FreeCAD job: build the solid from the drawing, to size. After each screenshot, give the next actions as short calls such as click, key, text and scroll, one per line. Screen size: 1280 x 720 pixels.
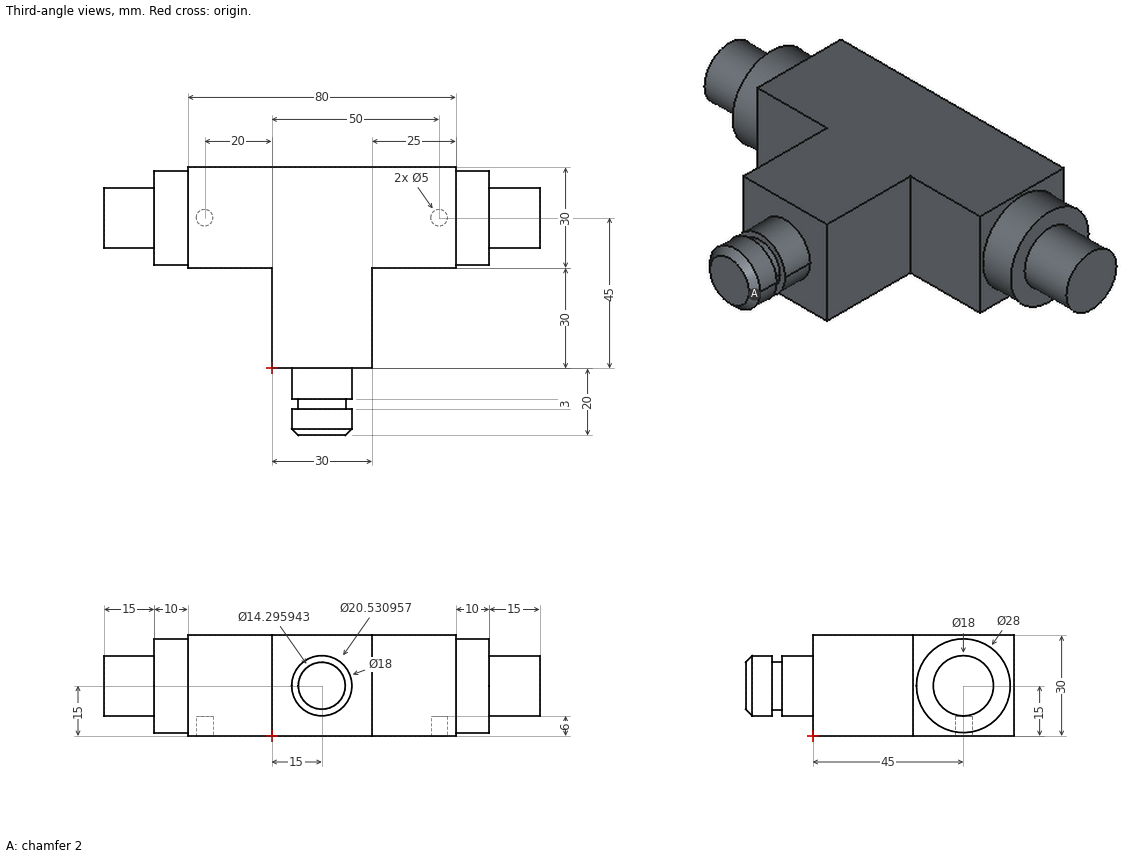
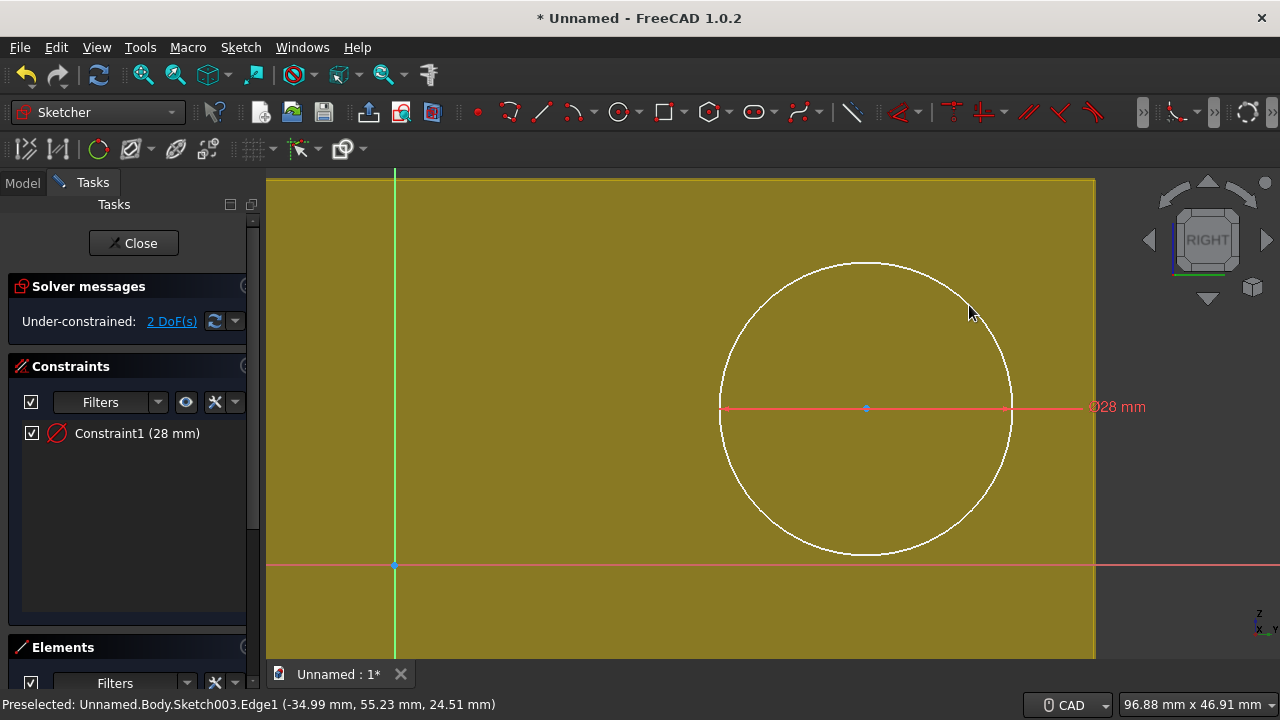
click(898, 112)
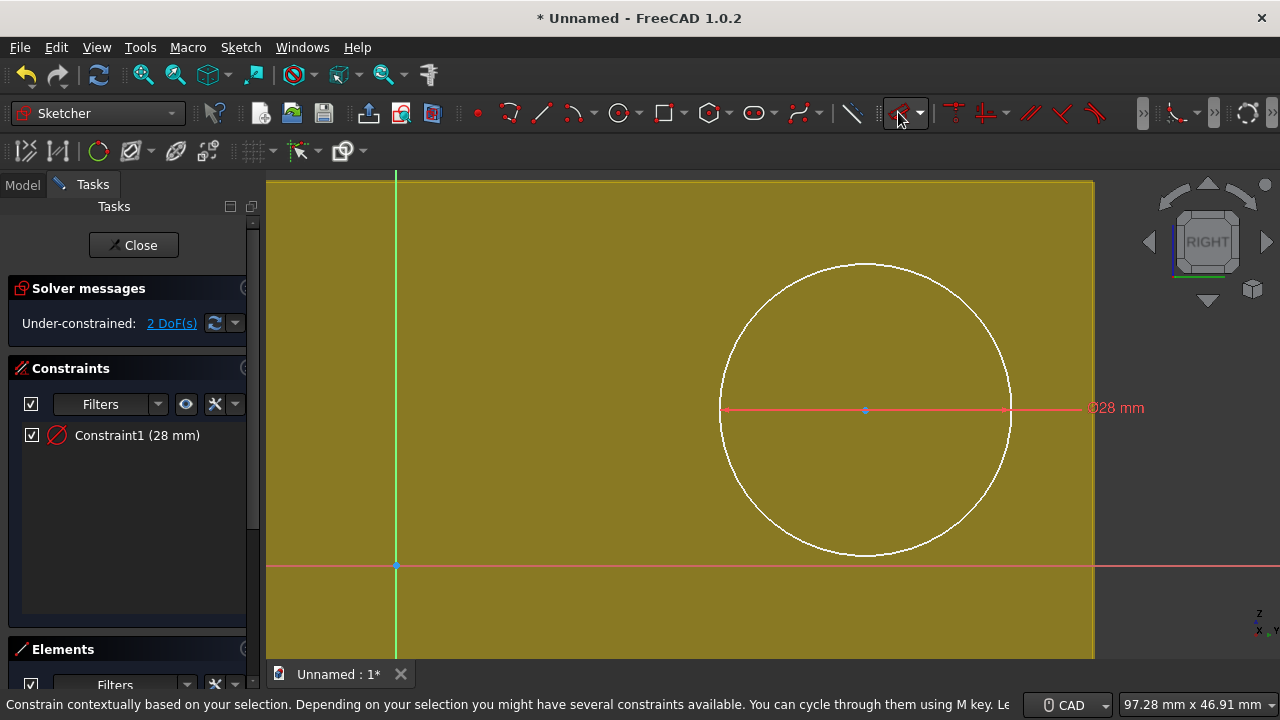
click(866, 410)
click(631, 600)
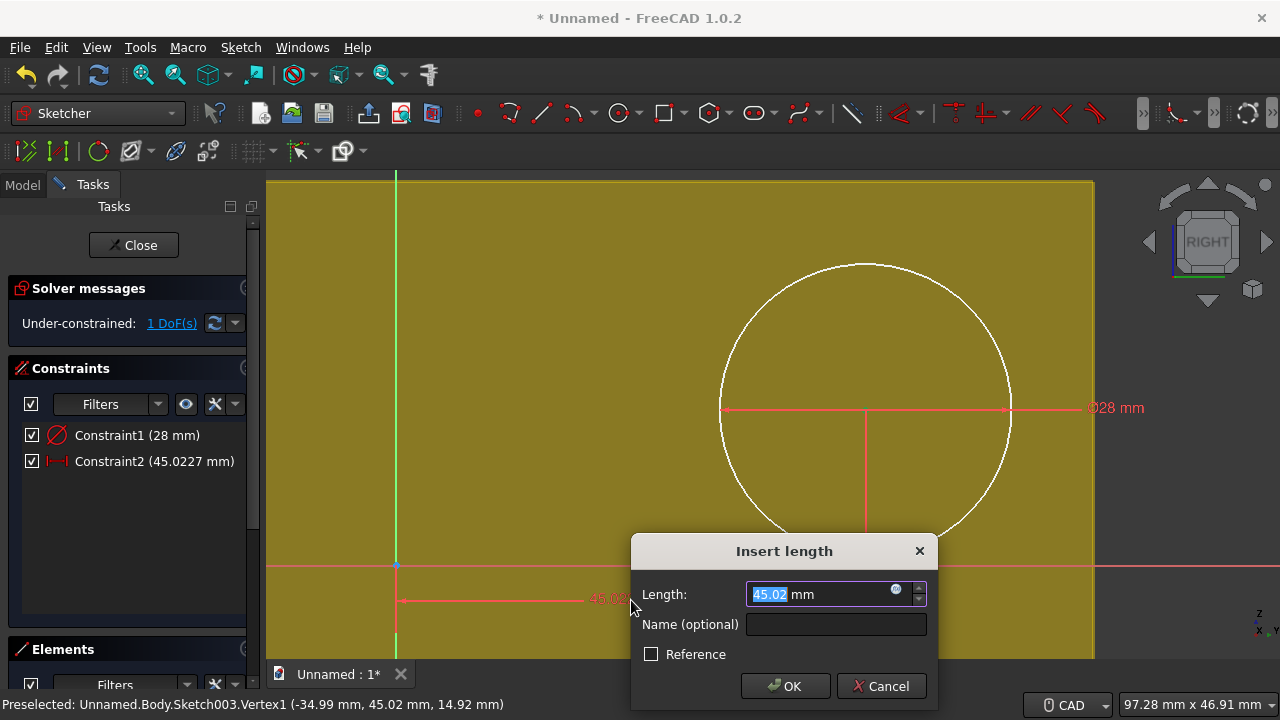
text(45)
key(Return)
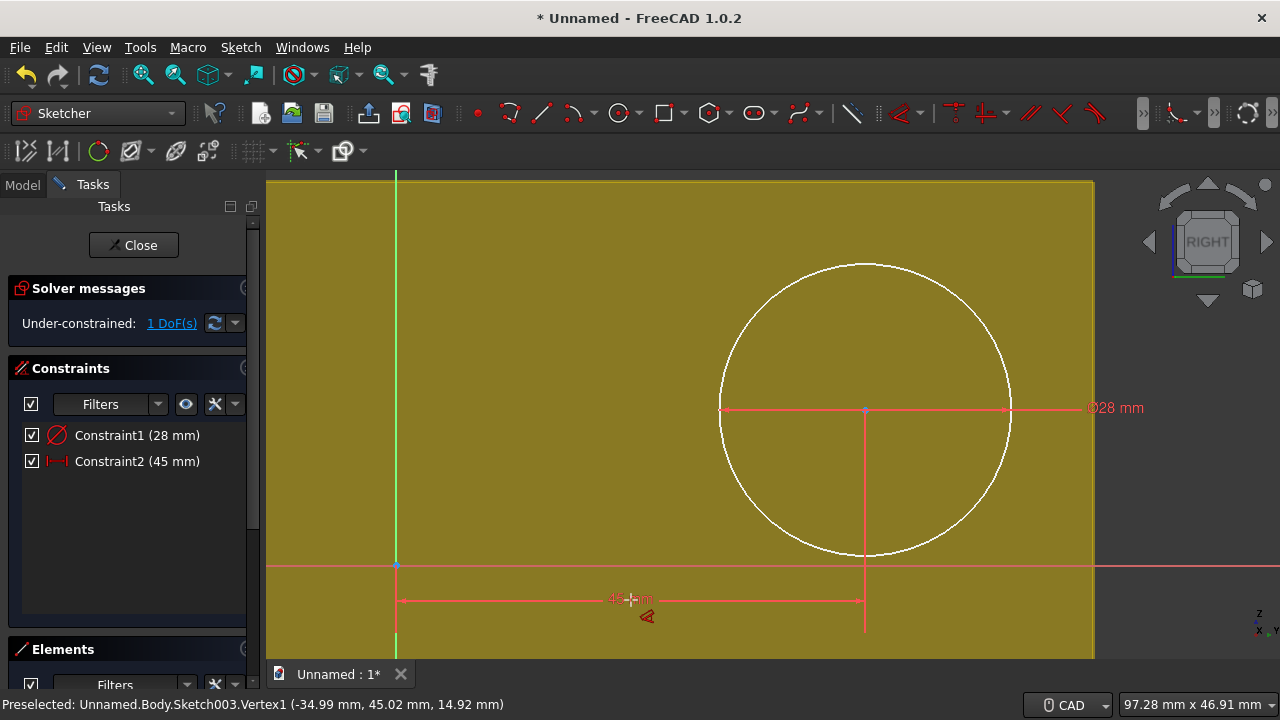
click(865, 410)
click(362, 488)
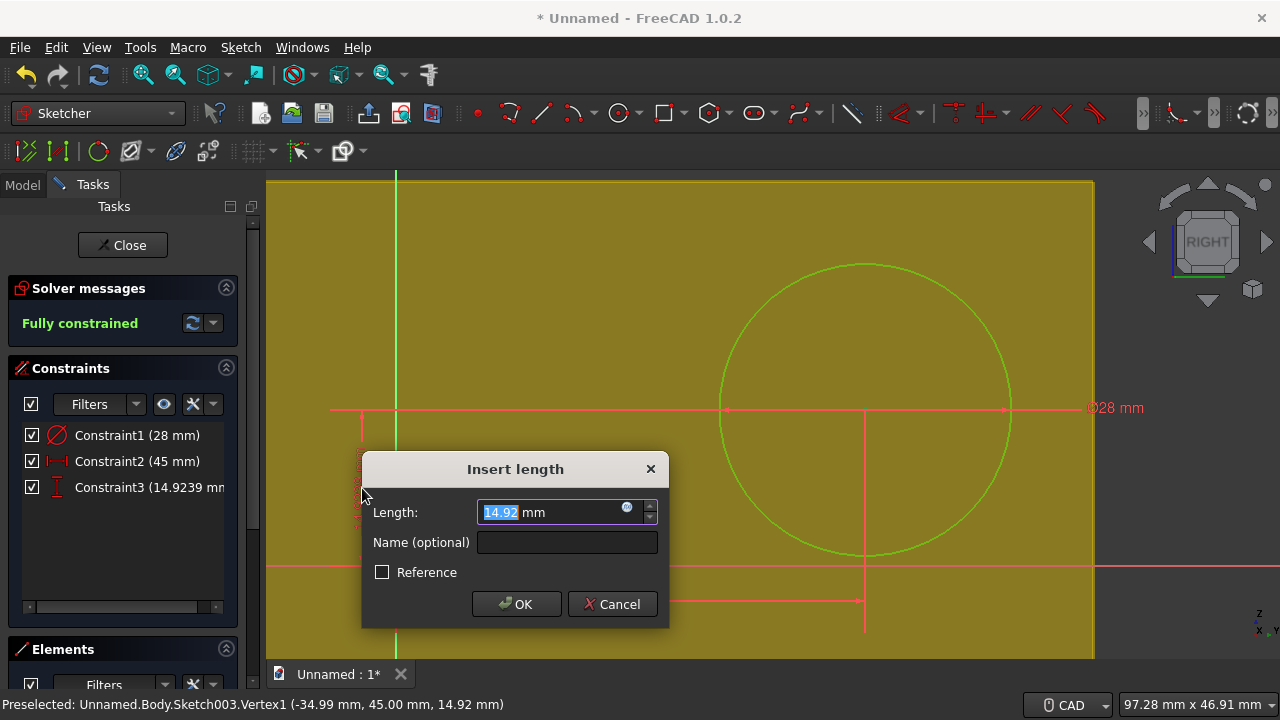
text(15)
key(Return)
key(Escape)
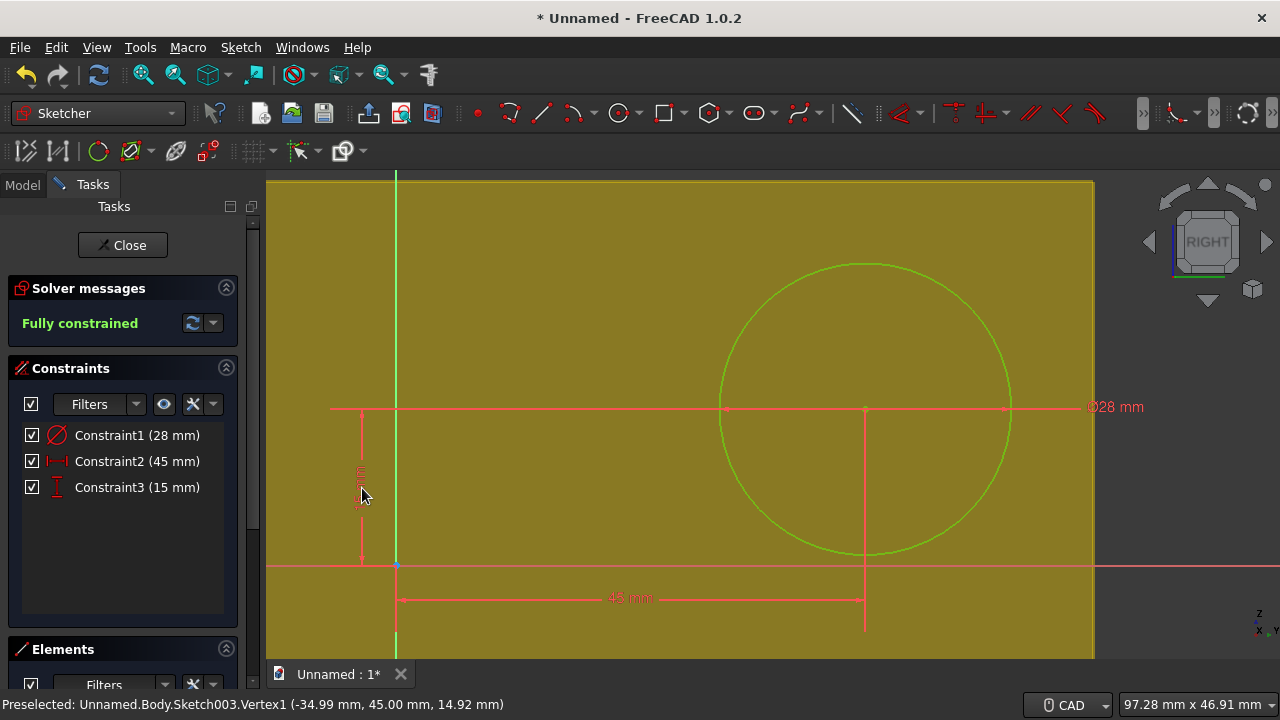
click(123, 245)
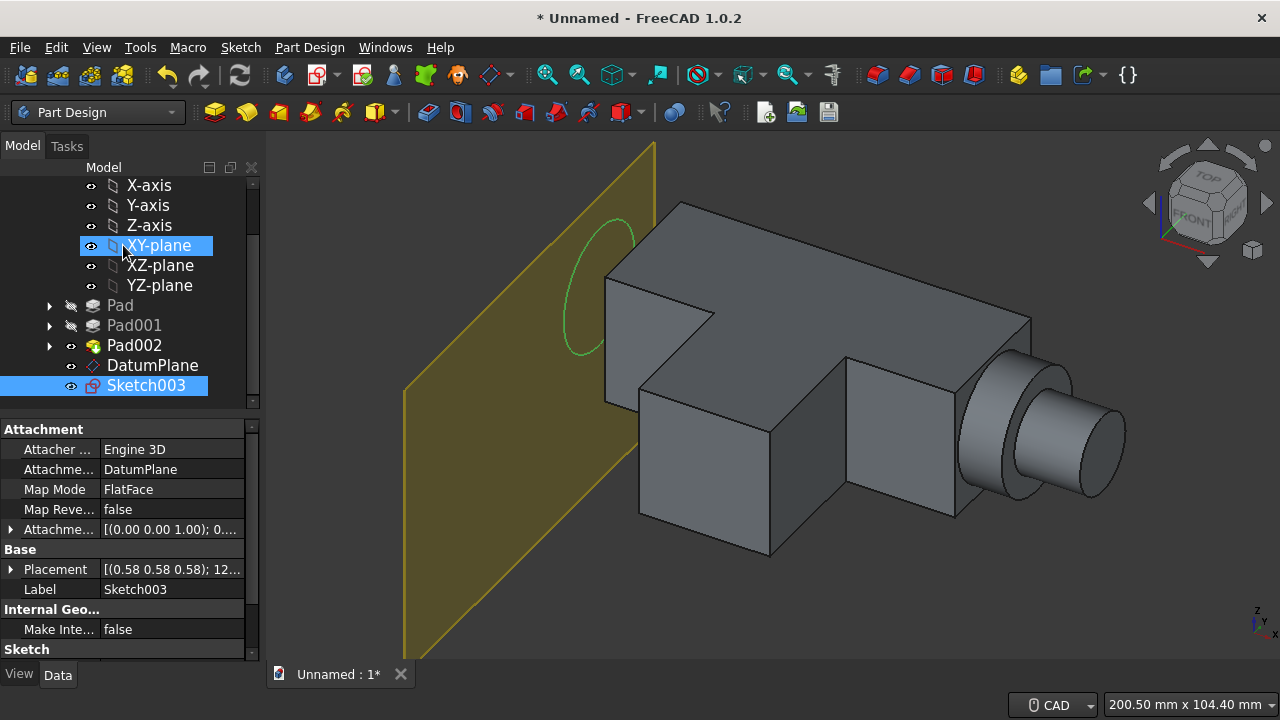
click(216, 112)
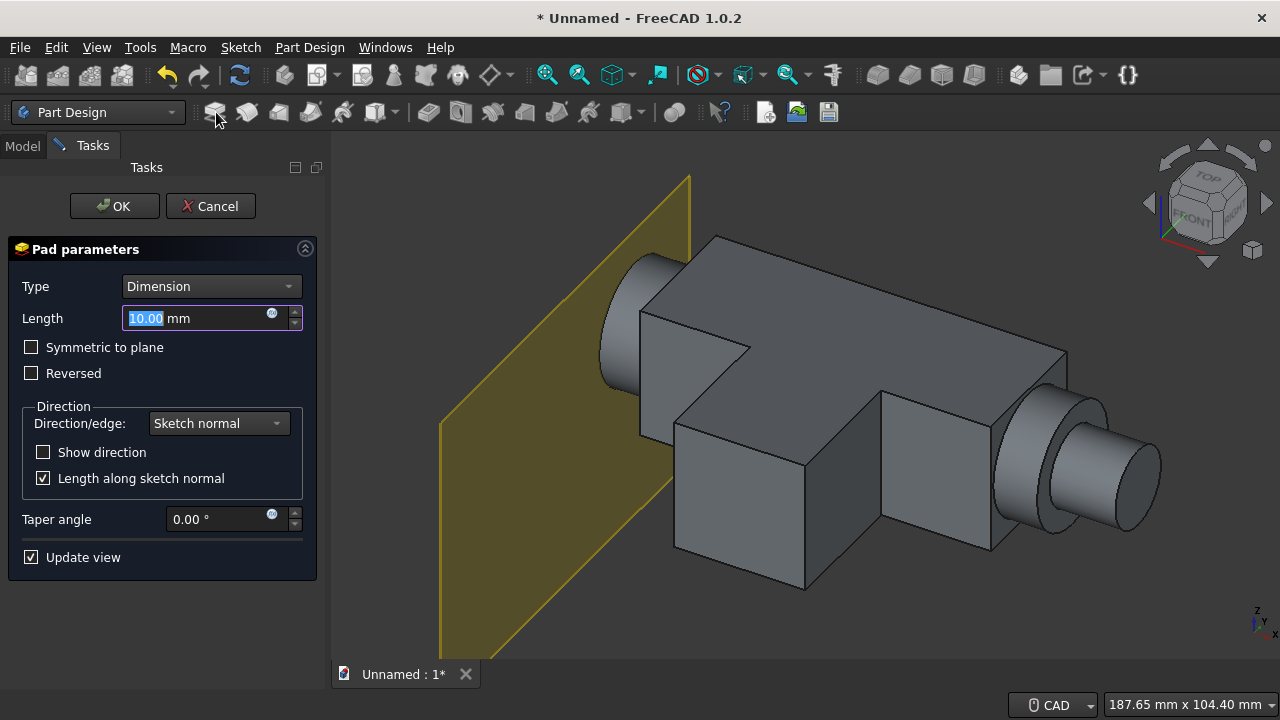
text(10)
key(Tab)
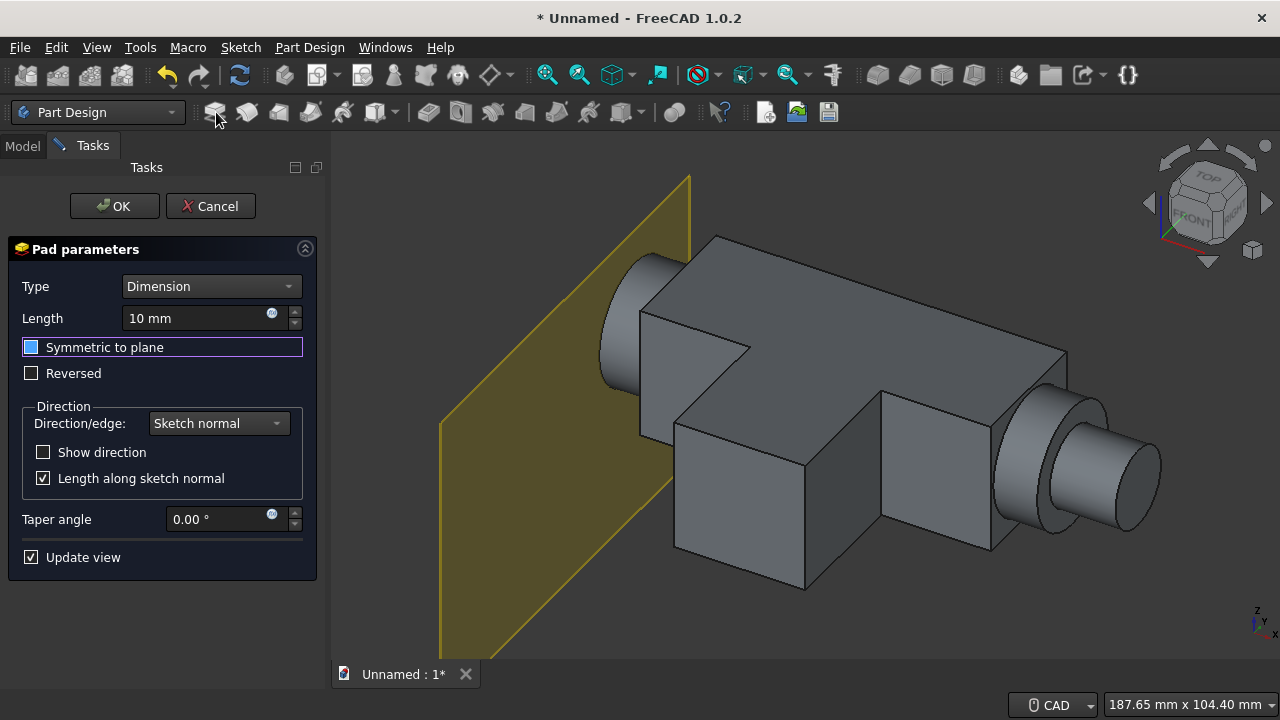
click(115, 206)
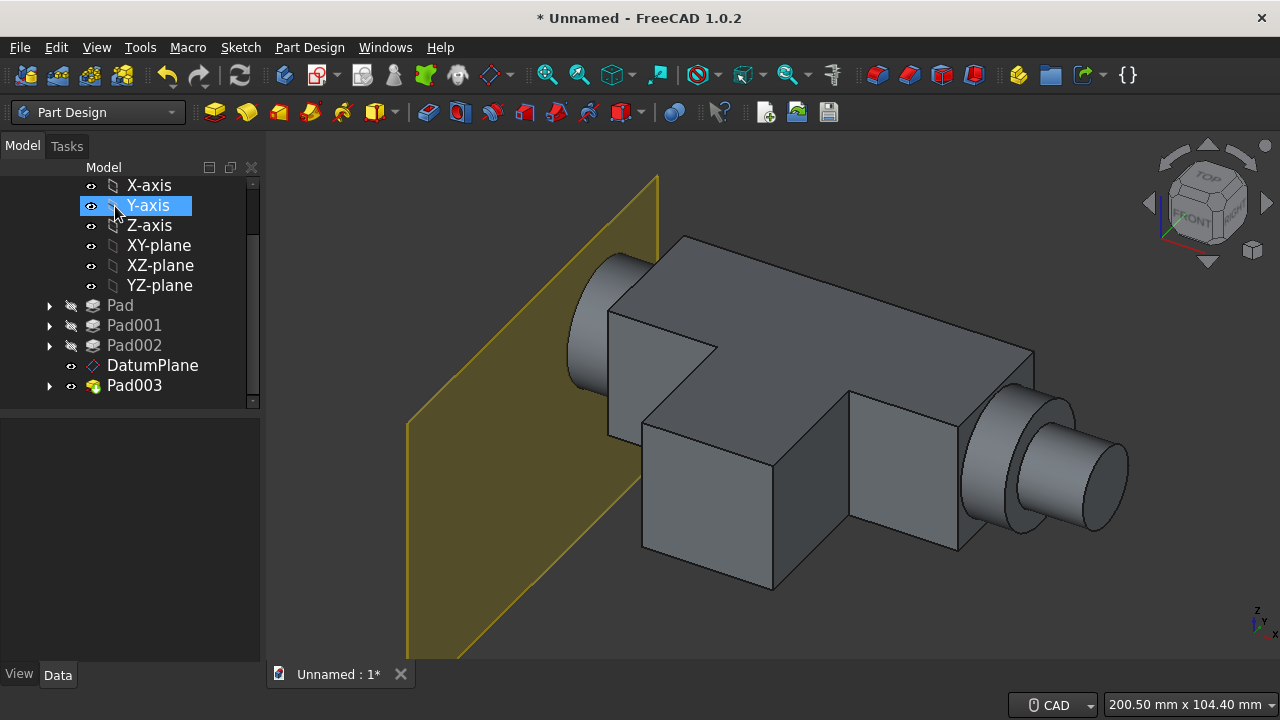
click(116, 366)
key(space)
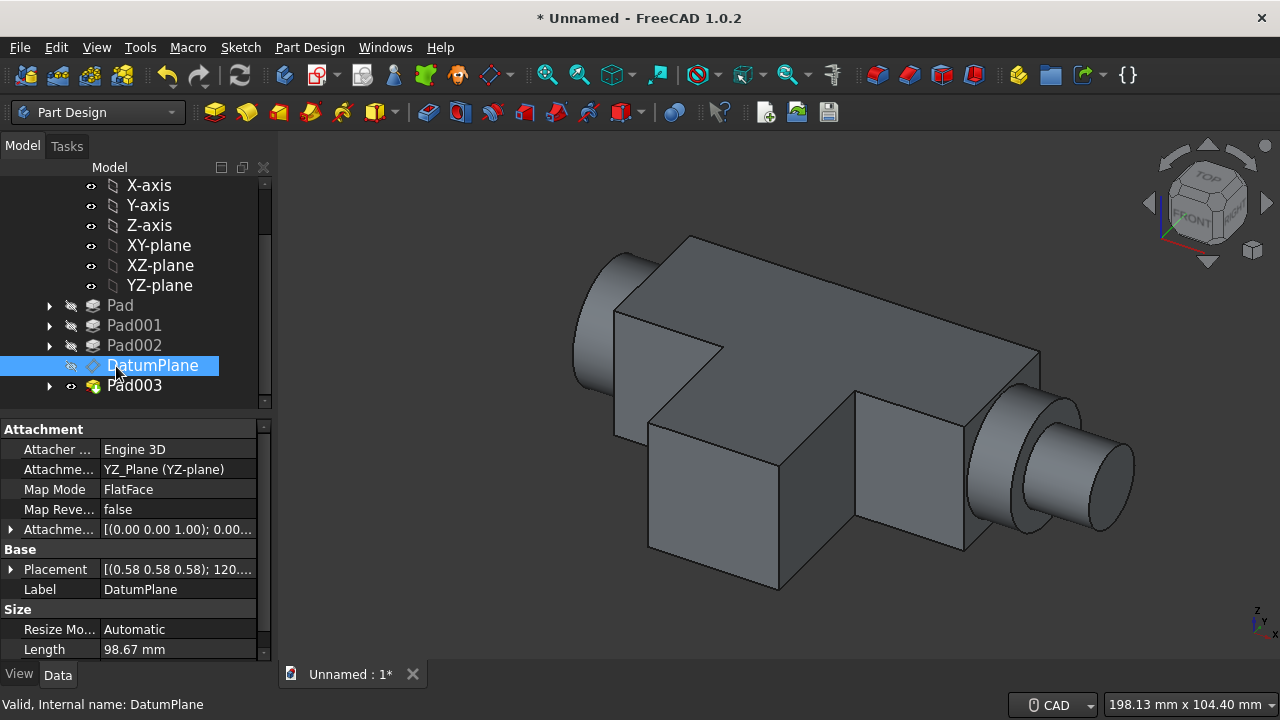
key(v)
key(f)